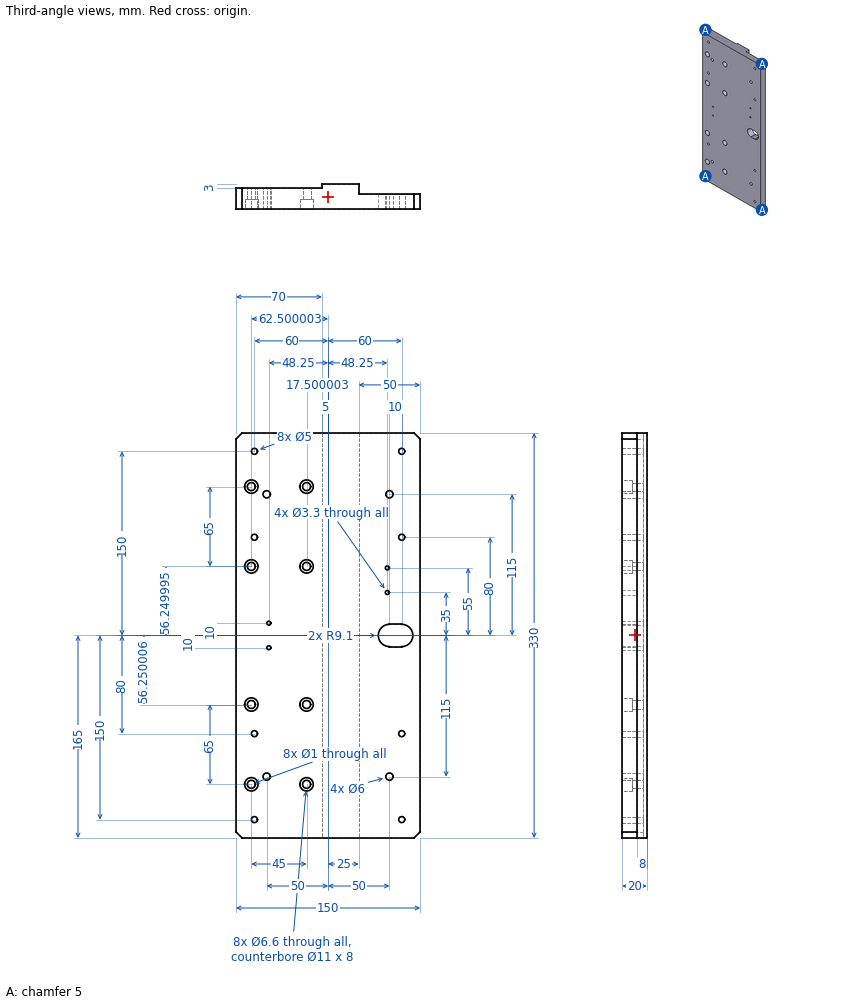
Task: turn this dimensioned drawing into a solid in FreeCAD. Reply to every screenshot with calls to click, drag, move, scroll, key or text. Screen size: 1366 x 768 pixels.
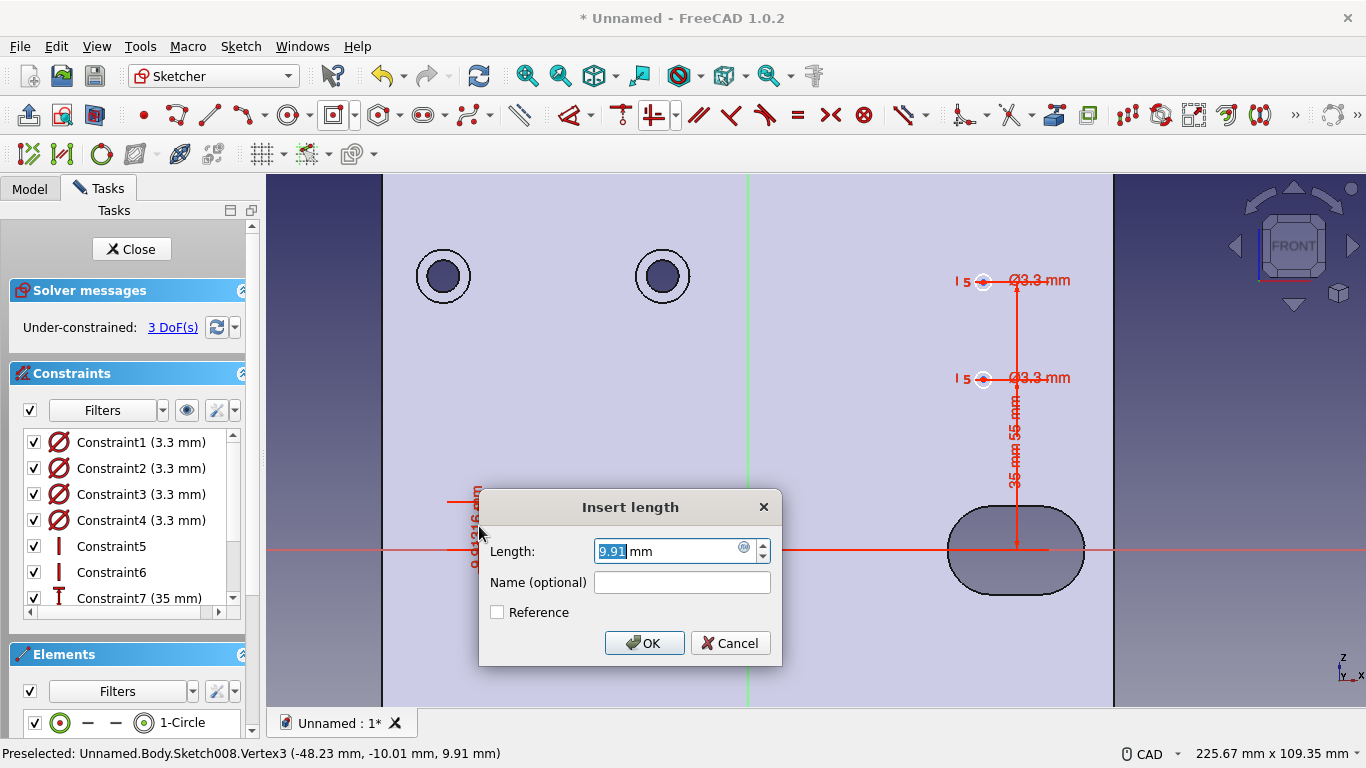
text(10)
key(Return)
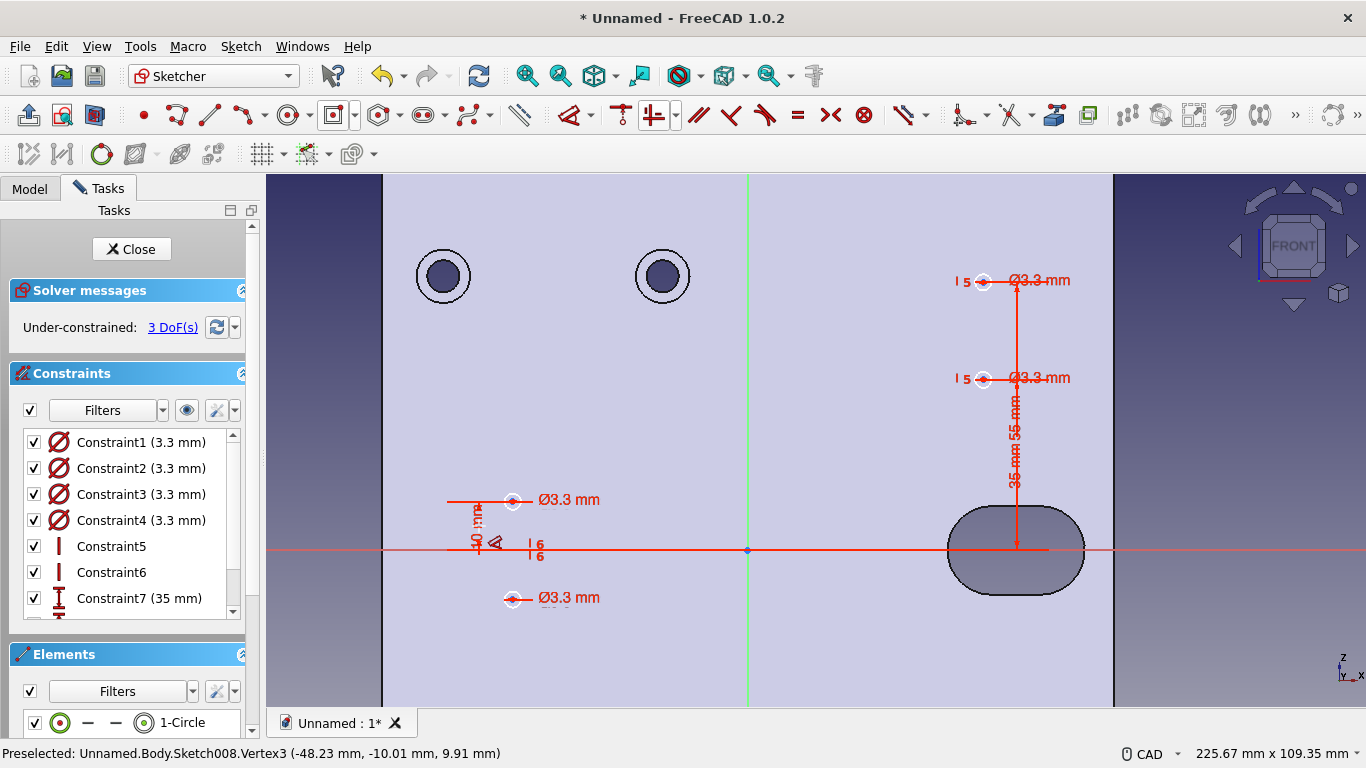
click(513, 600)
click(479, 575)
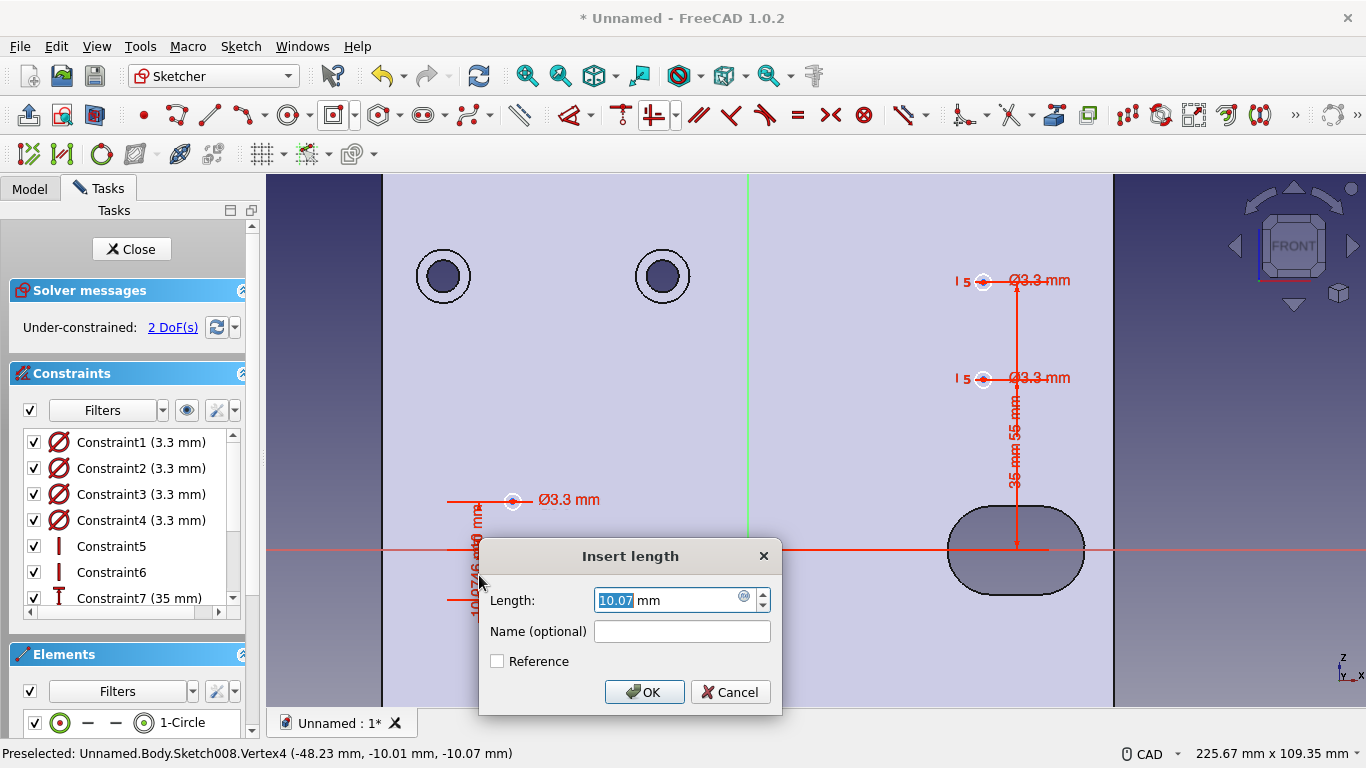
text(10)
key(Return)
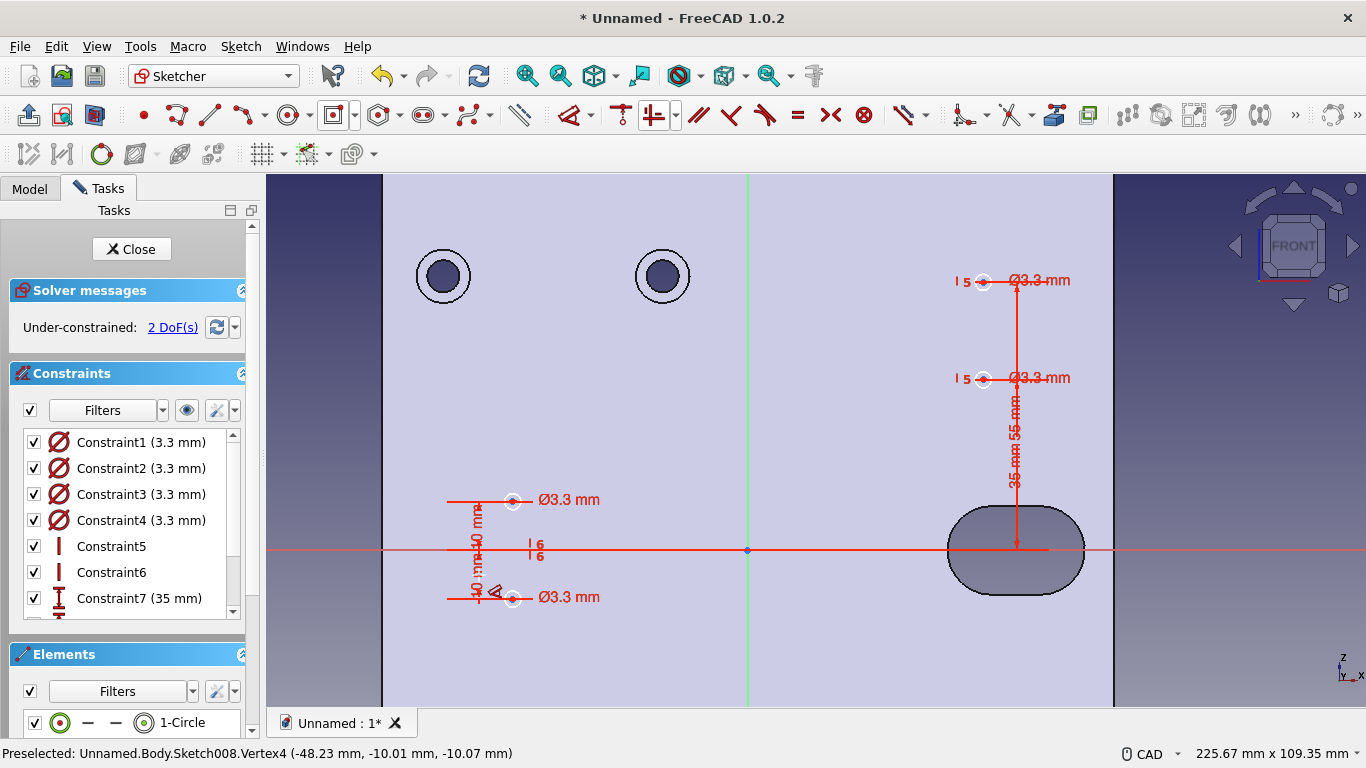
click(983, 380)
click(866, 584)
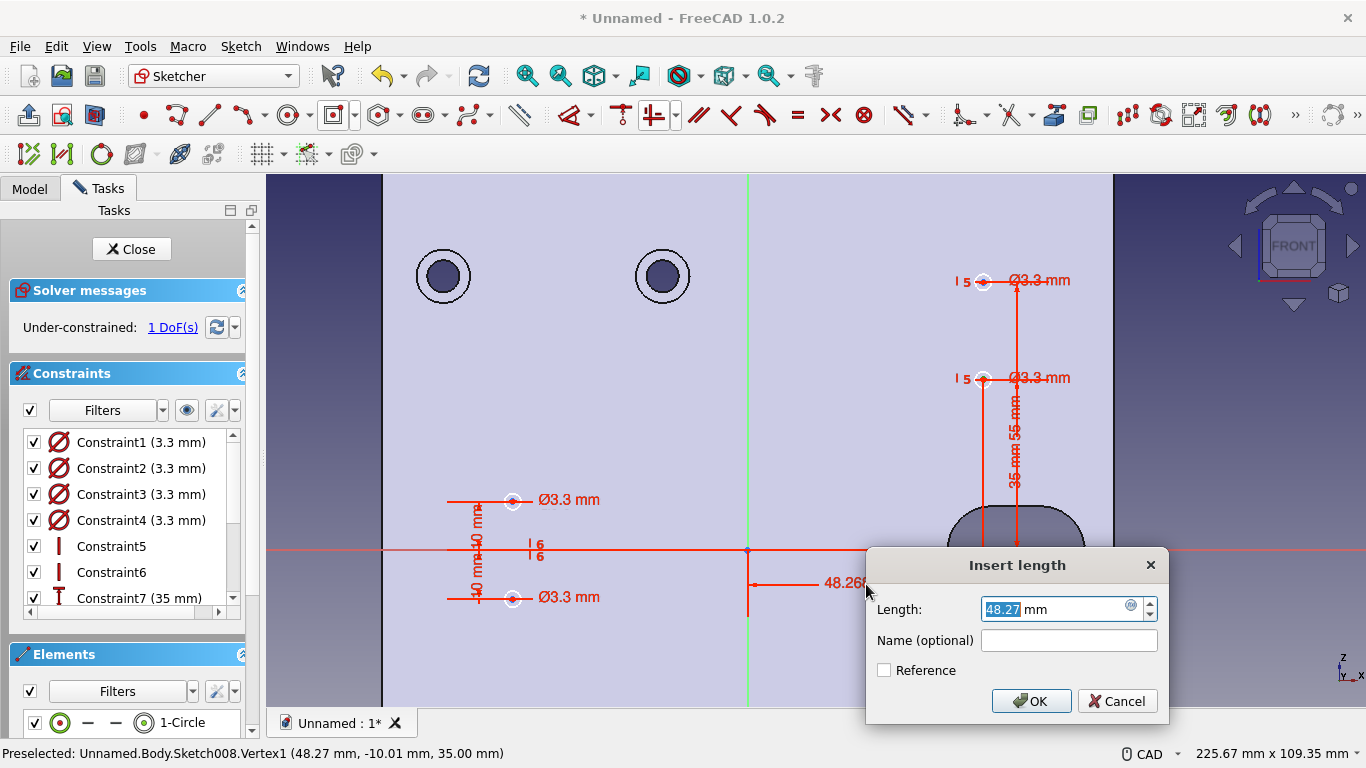
text(48.25)
key(Return)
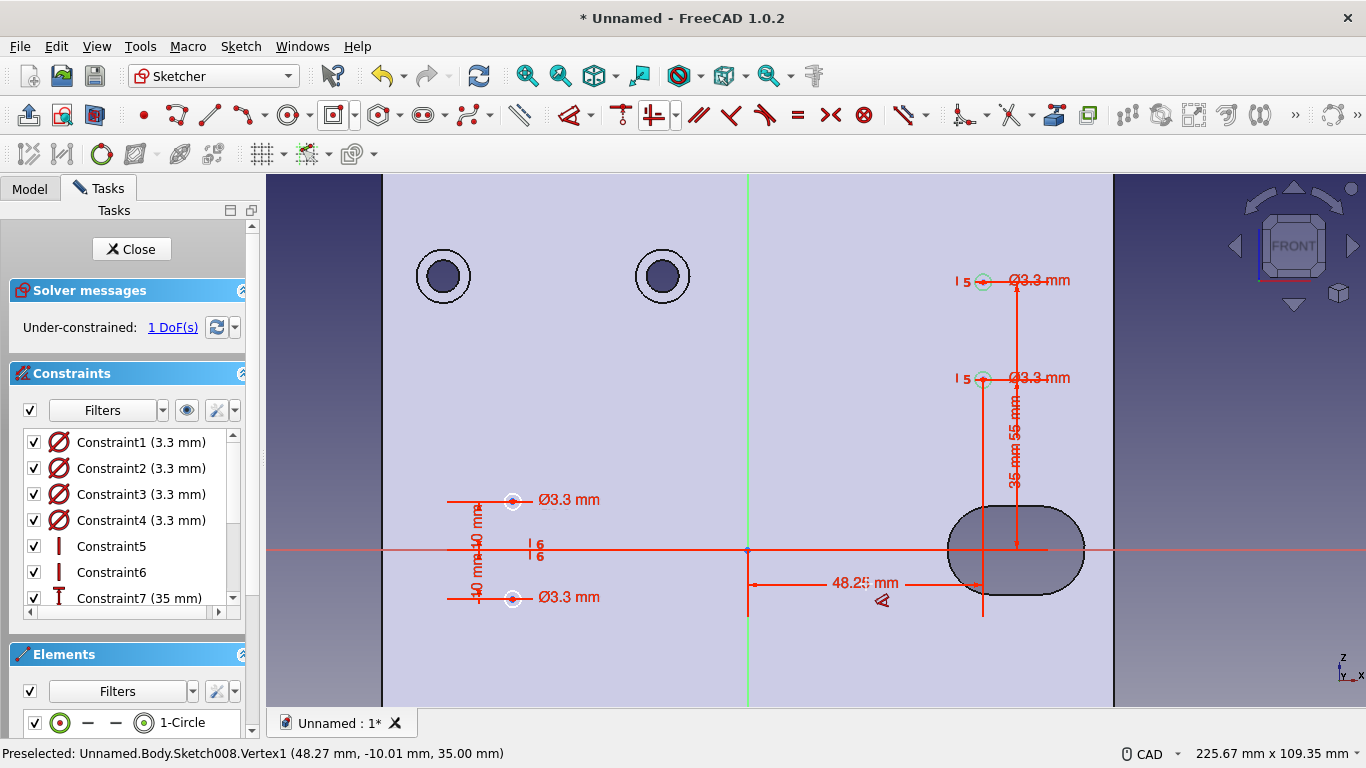
click(513, 502)
click(630, 584)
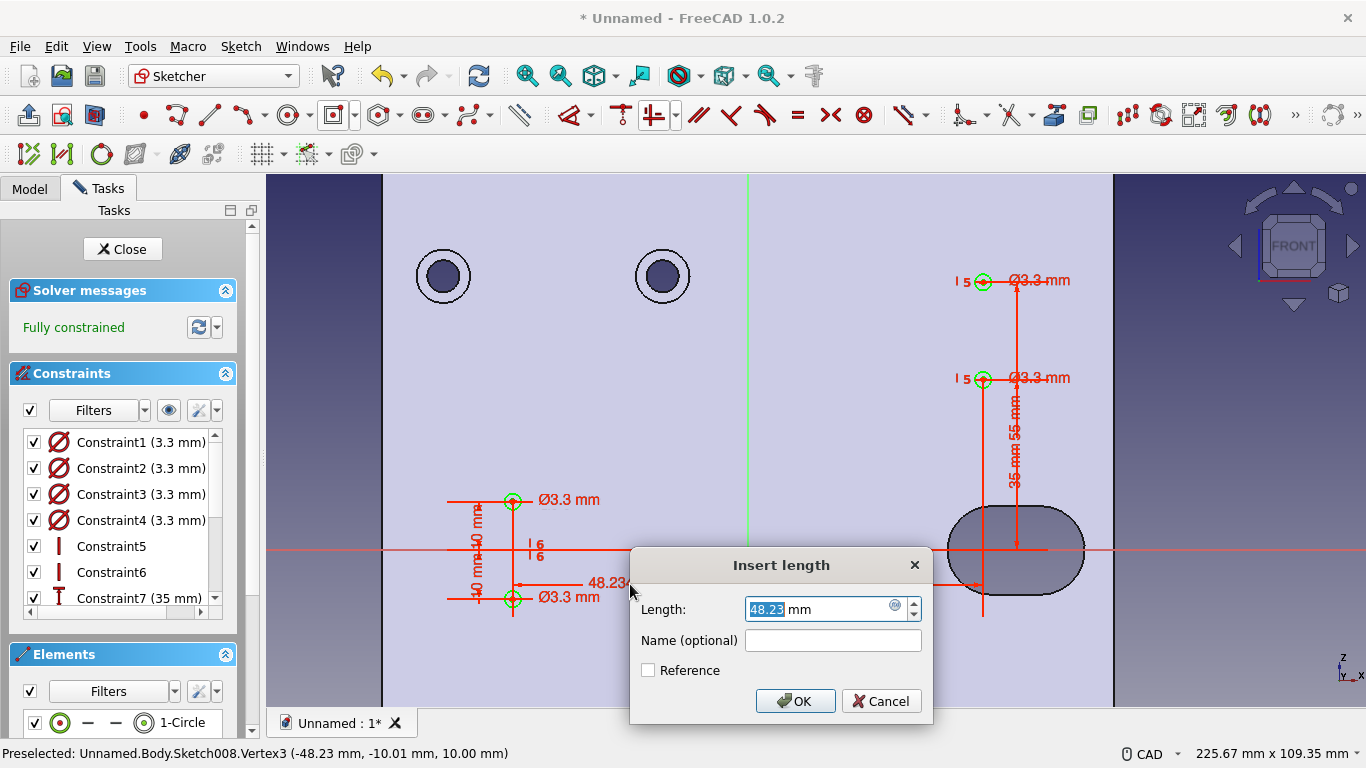
text(48.25)
key(Return)
key(Escape)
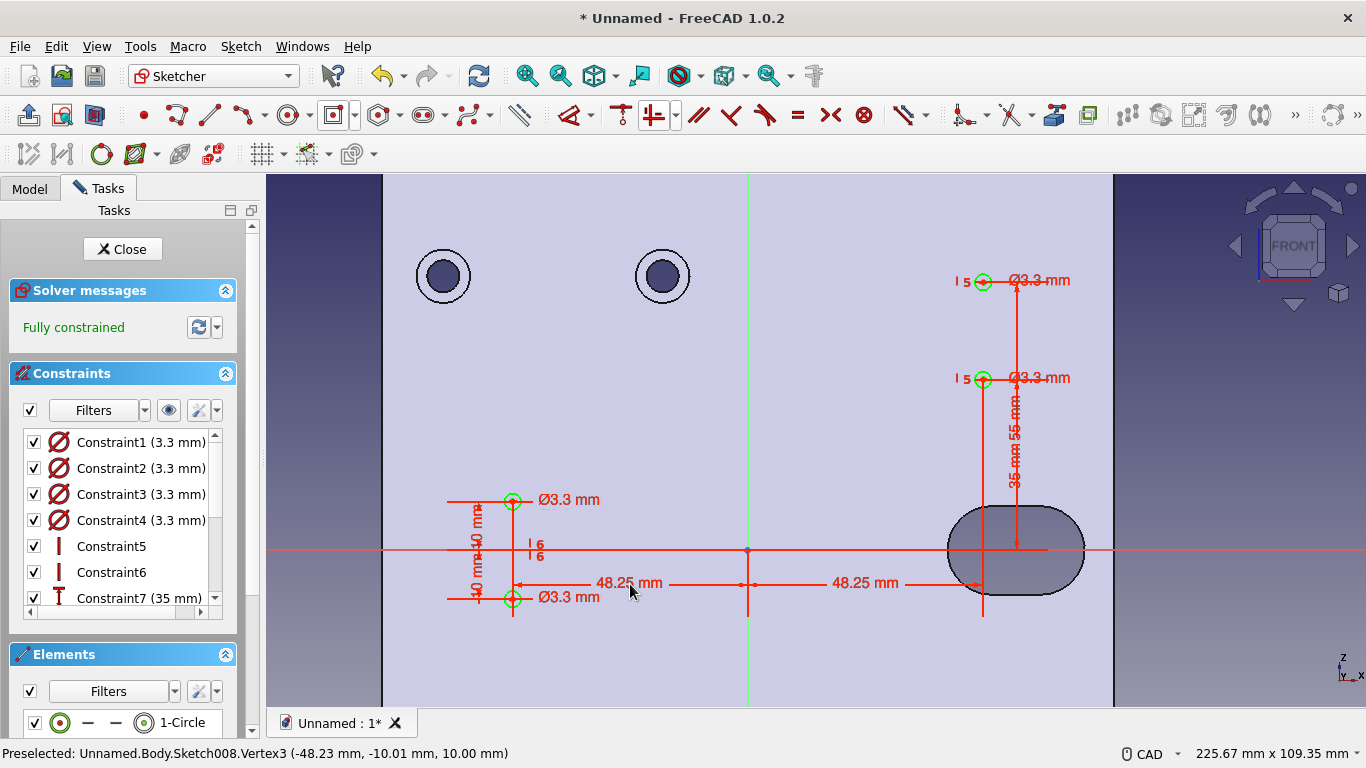
click(123, 249)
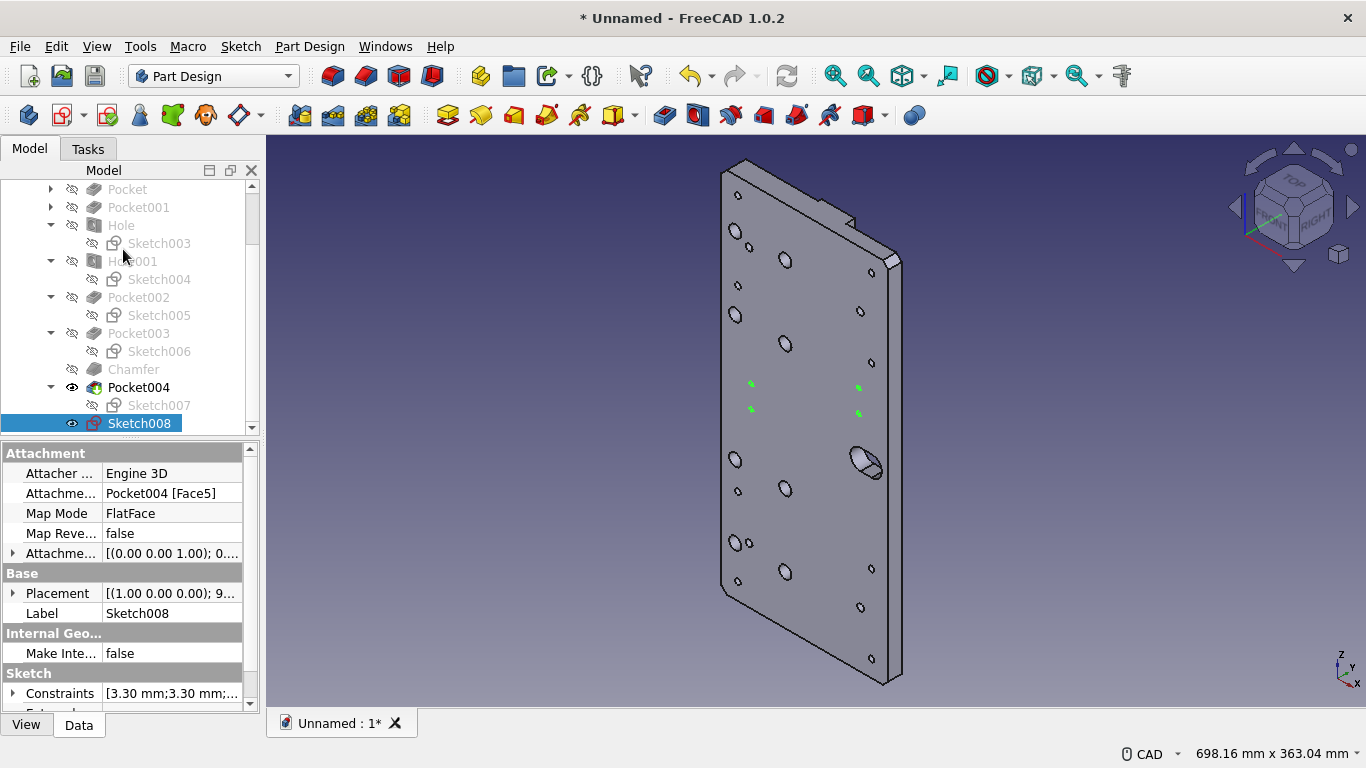
click(698, 116)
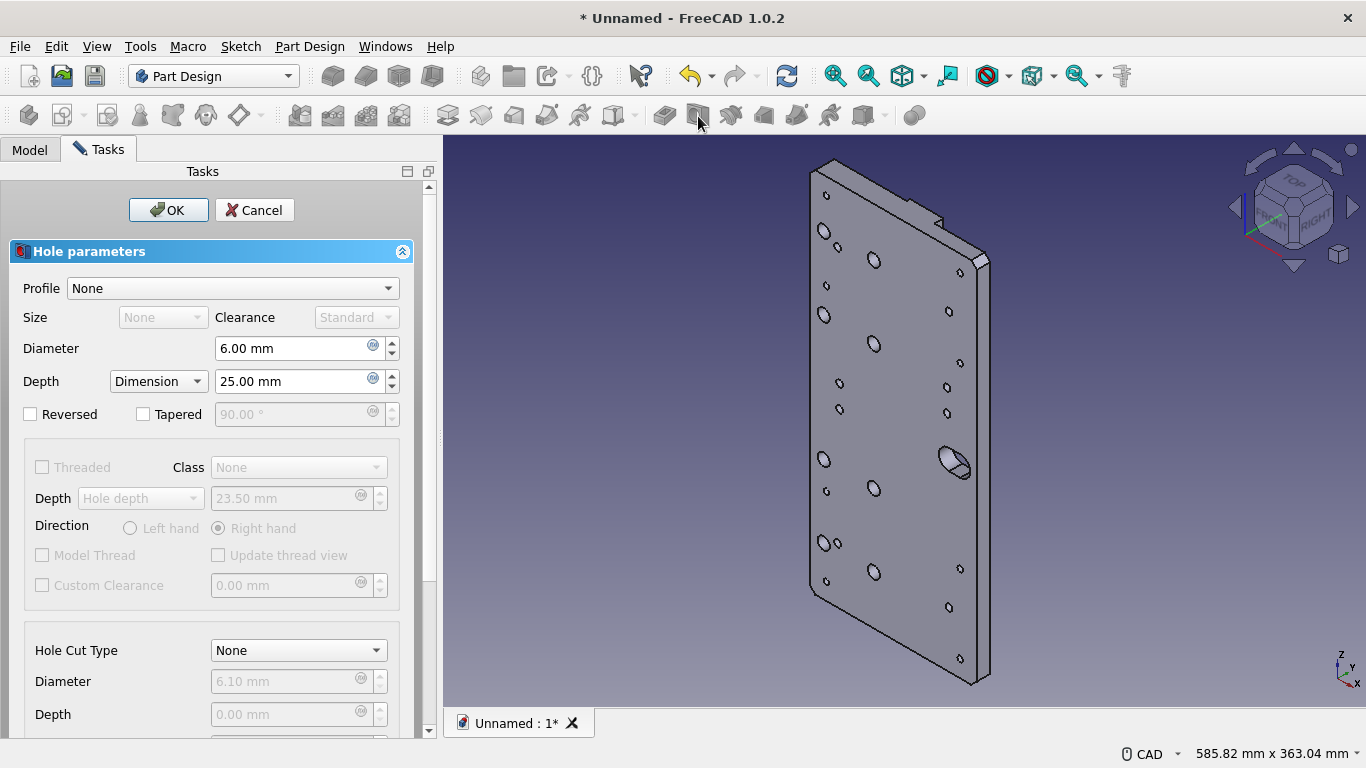
triple_click(300, 348)